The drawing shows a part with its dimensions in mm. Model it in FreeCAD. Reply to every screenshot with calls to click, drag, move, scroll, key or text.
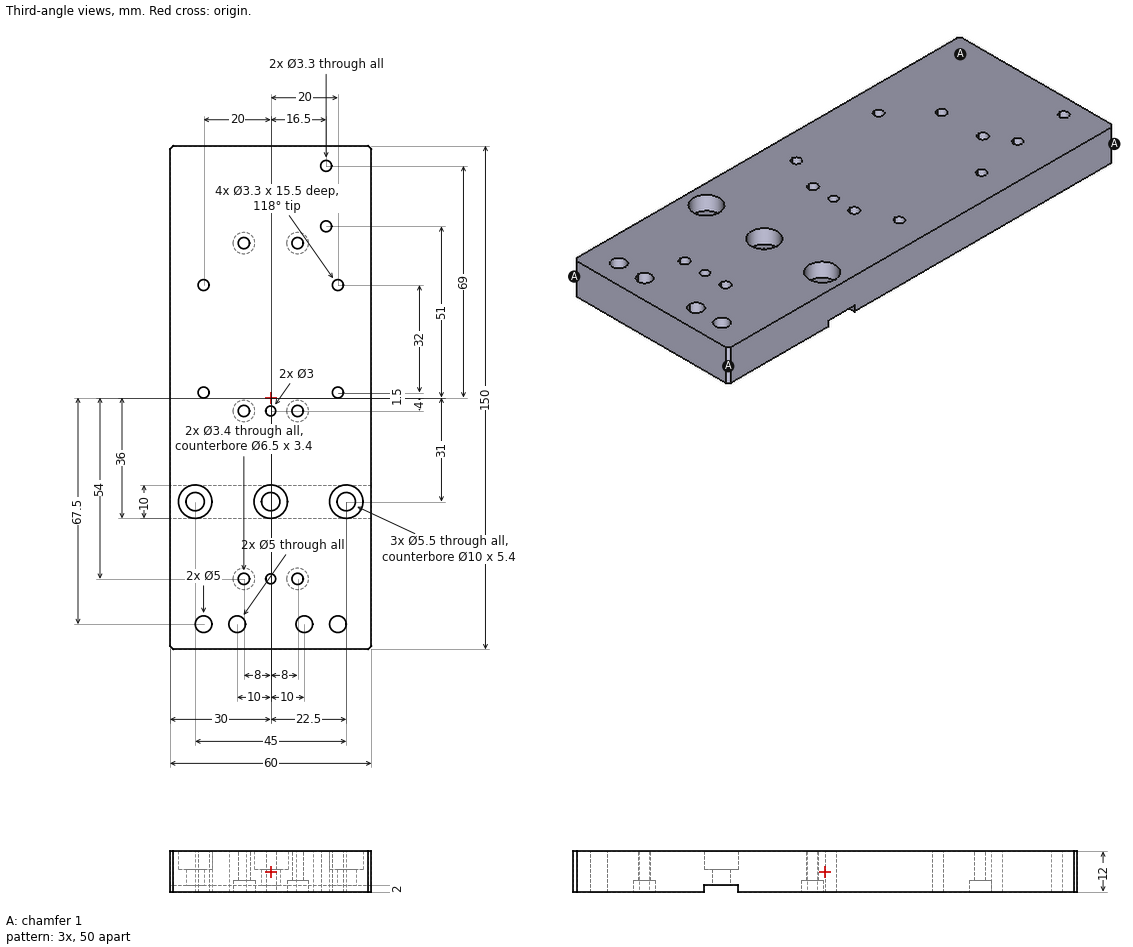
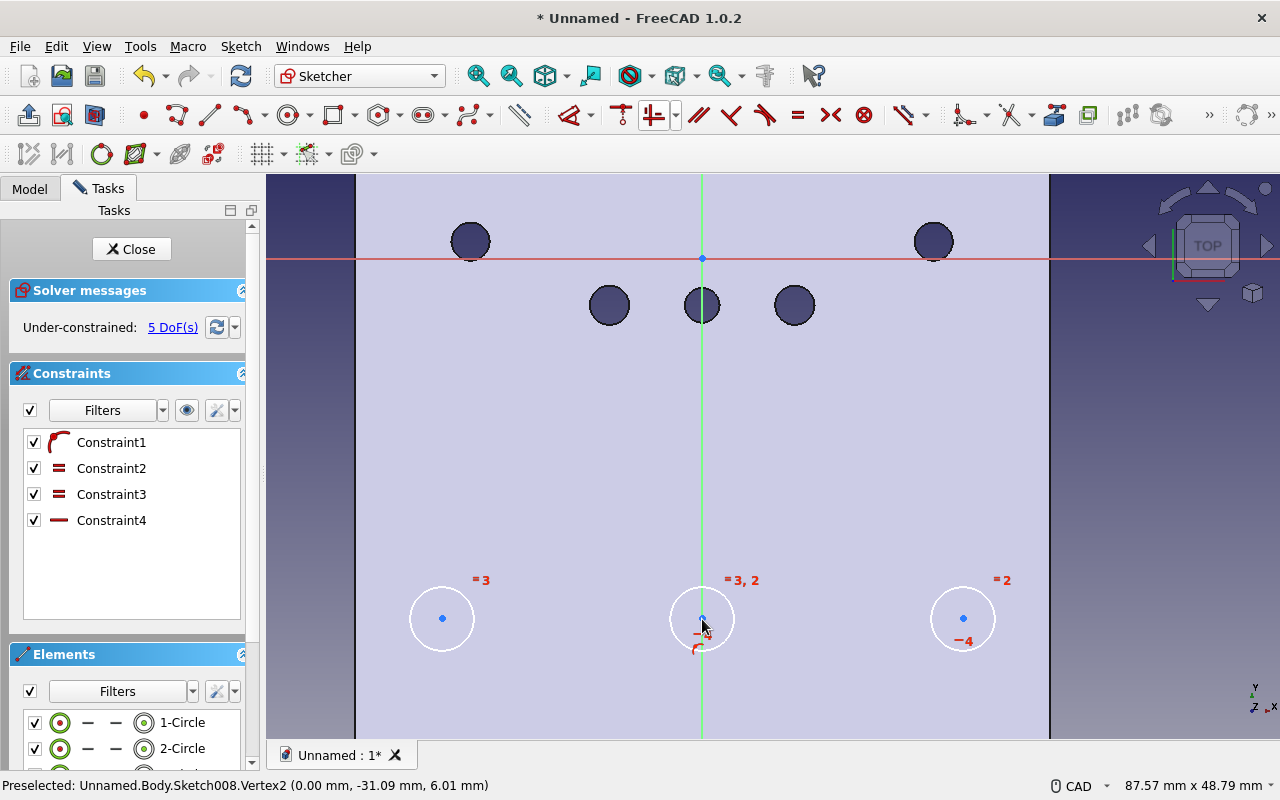
click(702, 619)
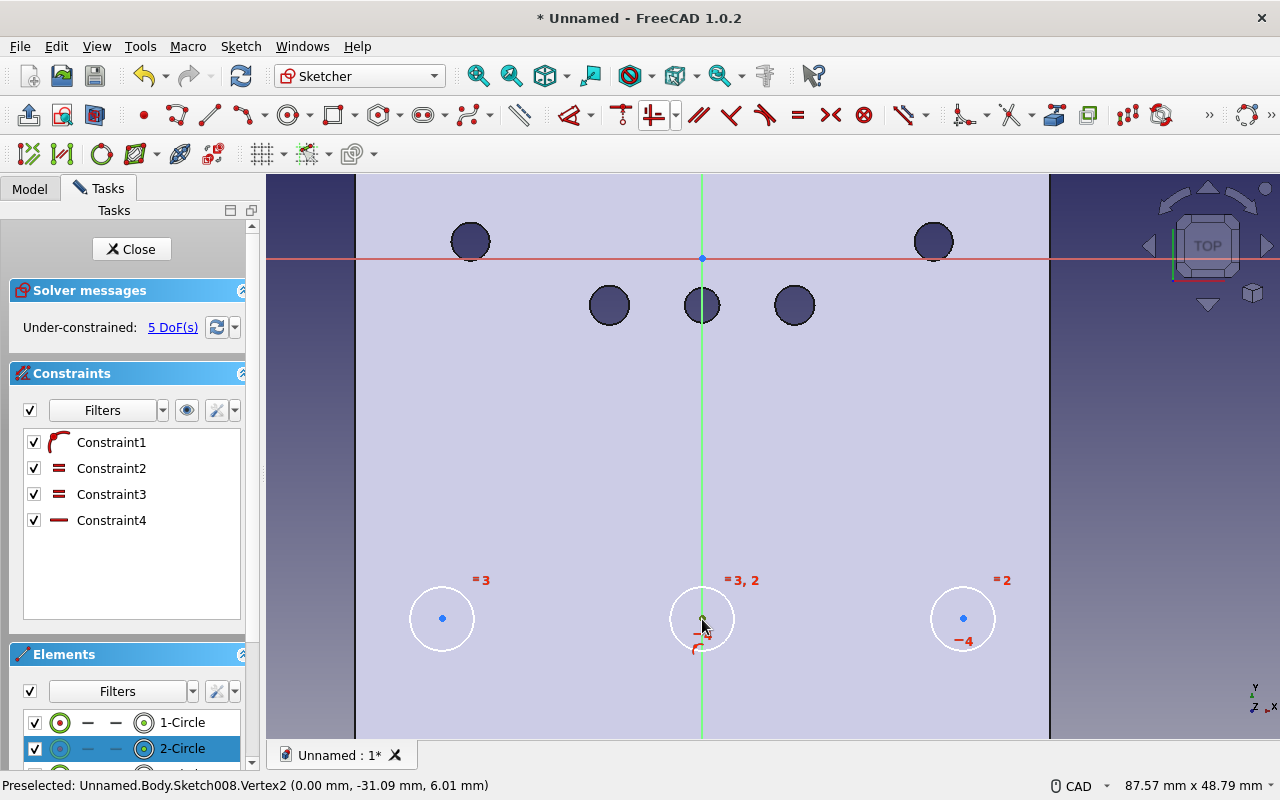
click(442, 619)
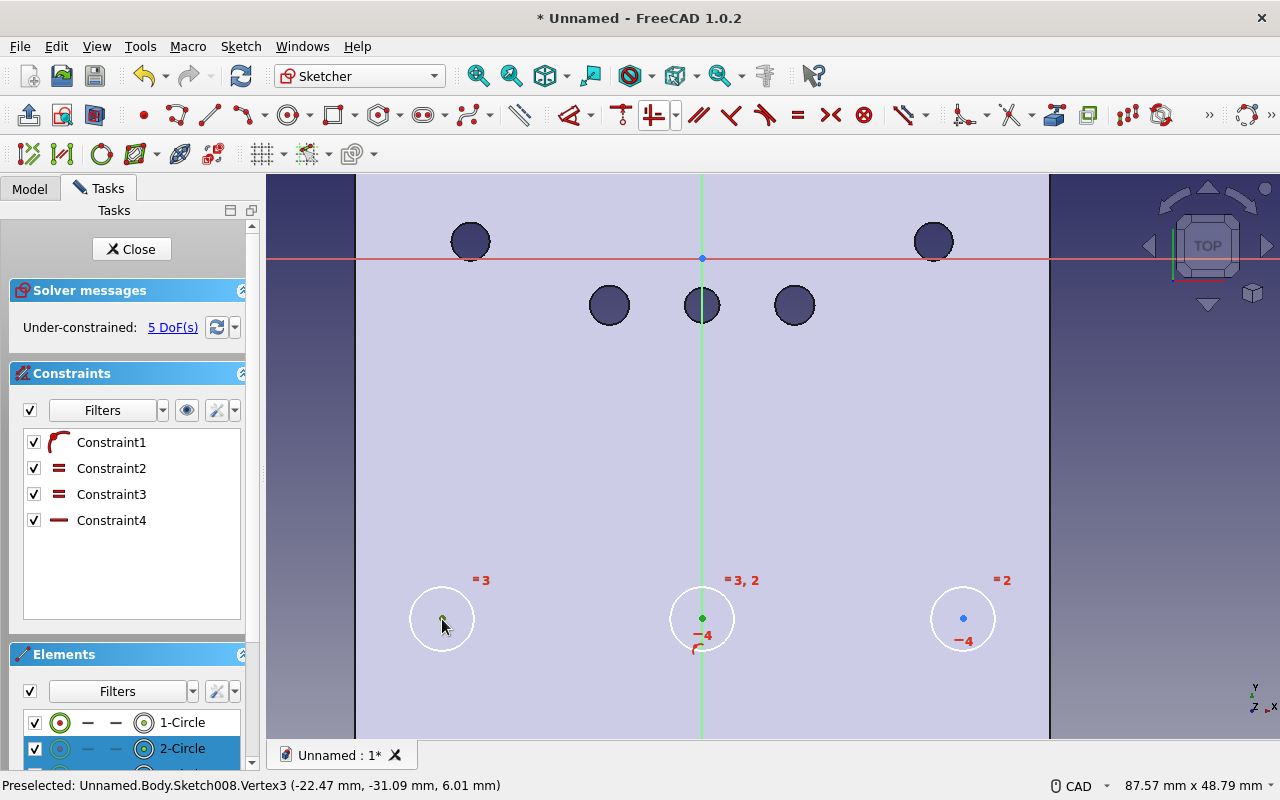
click(676, 116)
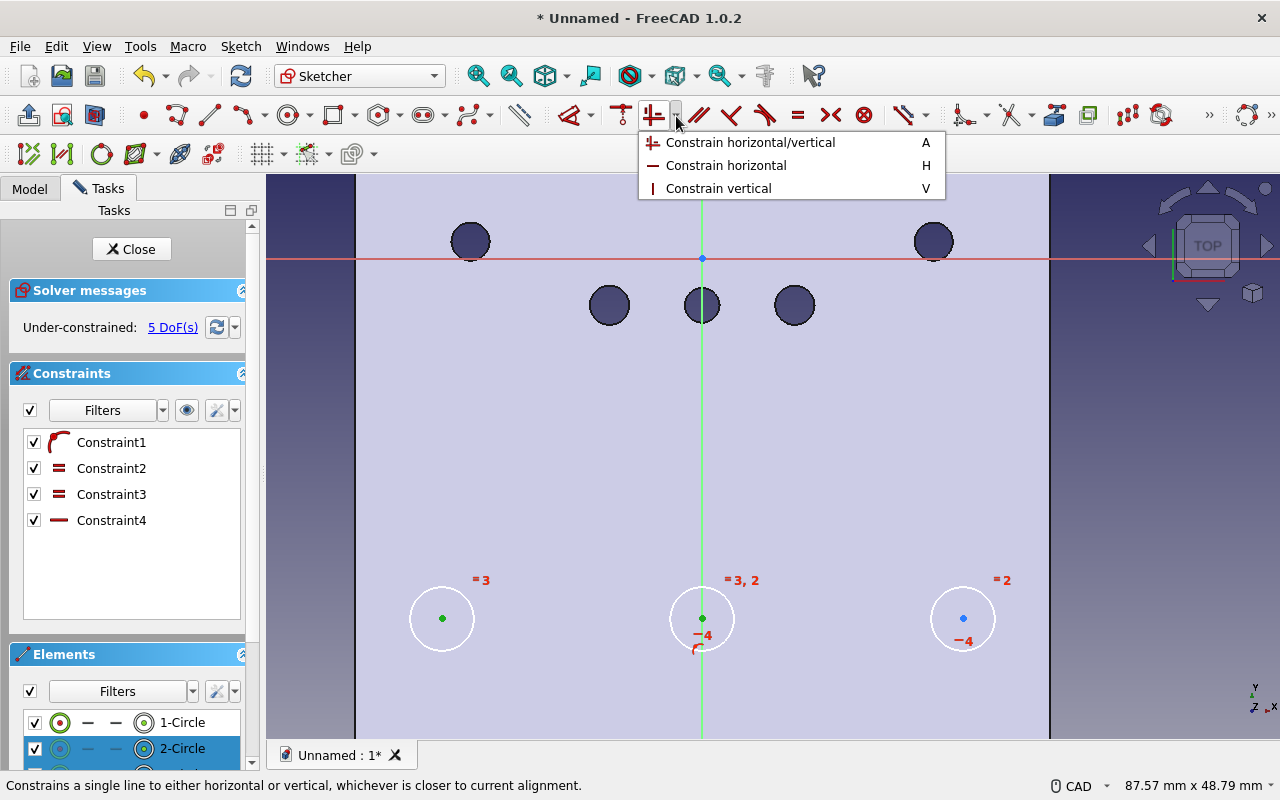
click(792, 166)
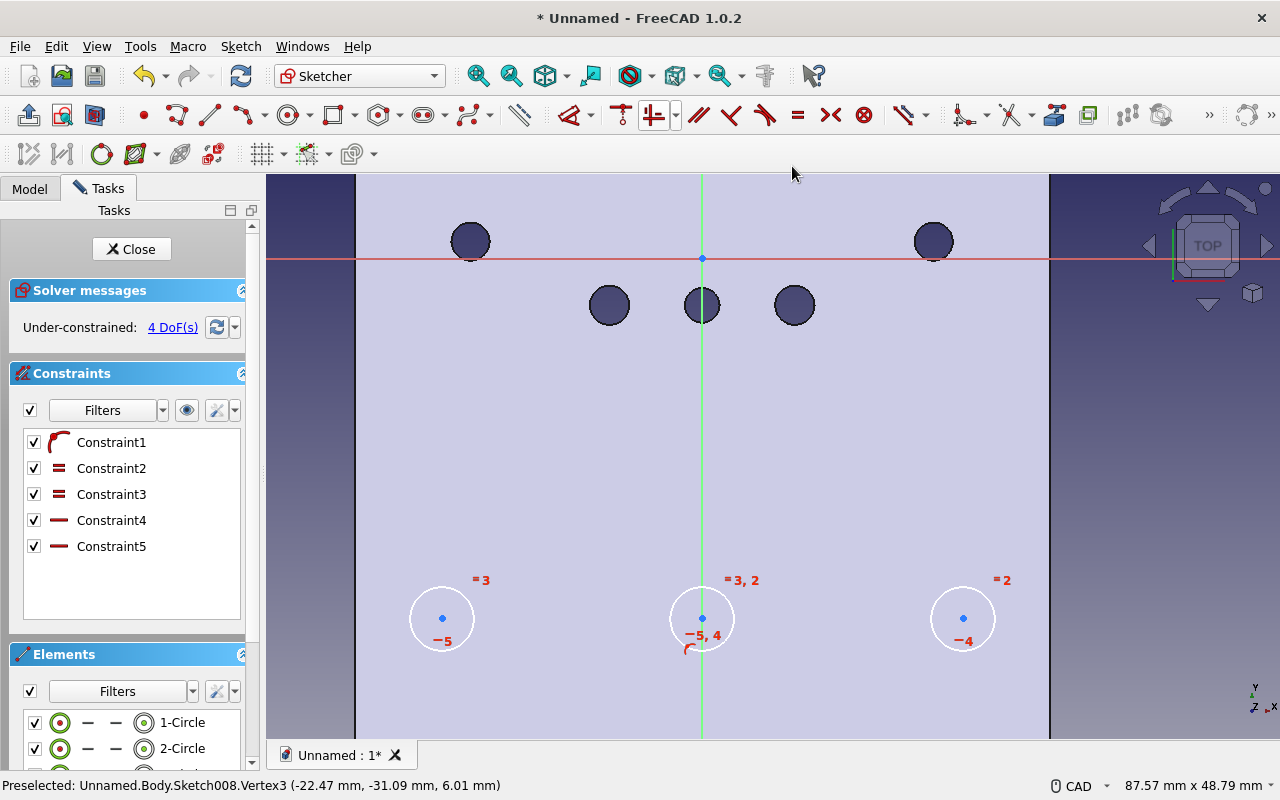
click(568, 116)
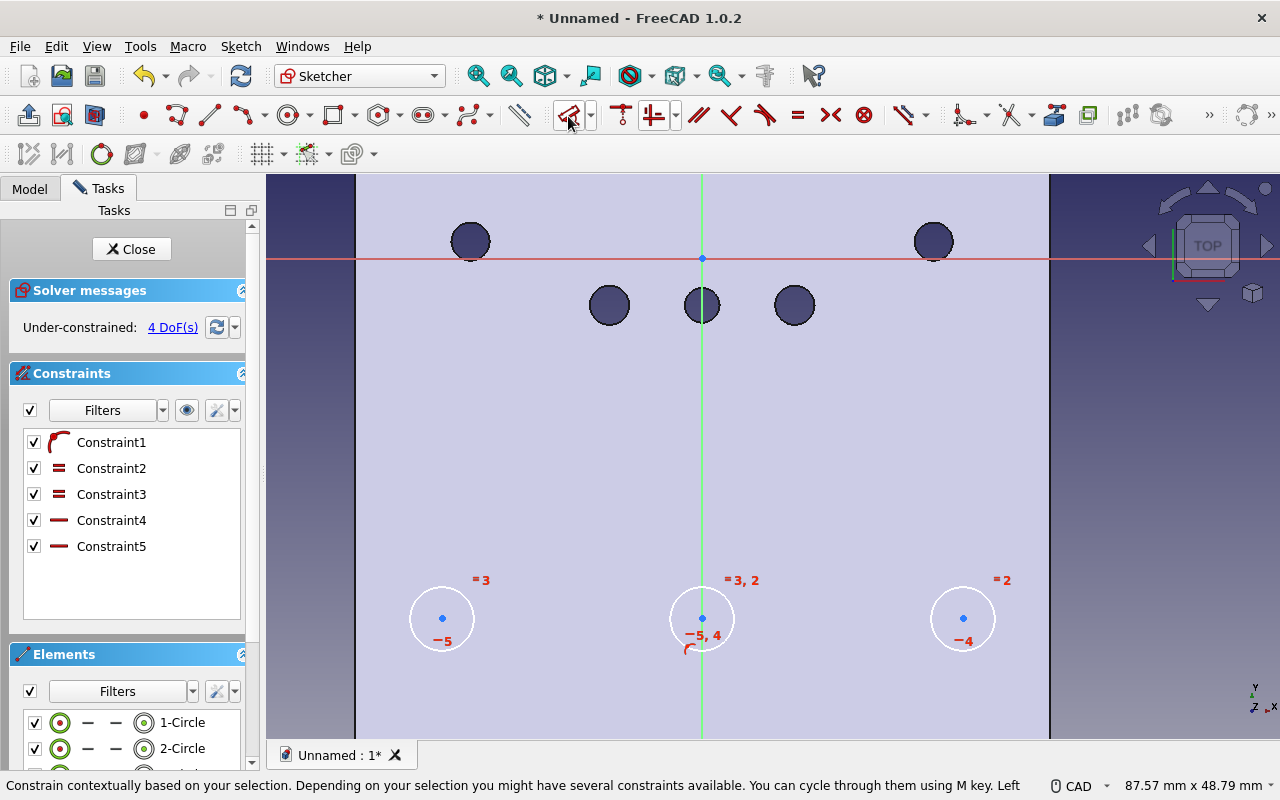
click(985, 596)
click(1007, 573)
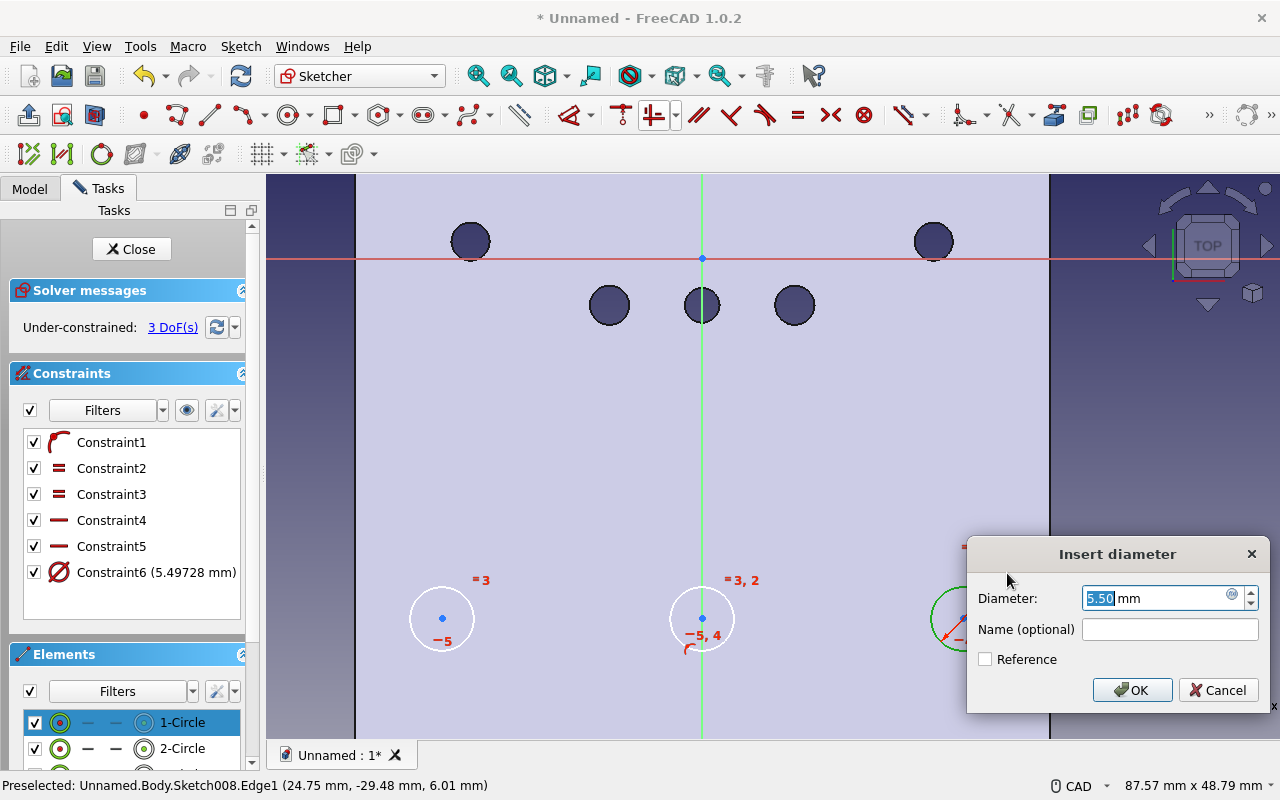
text(5.5)
key(Return)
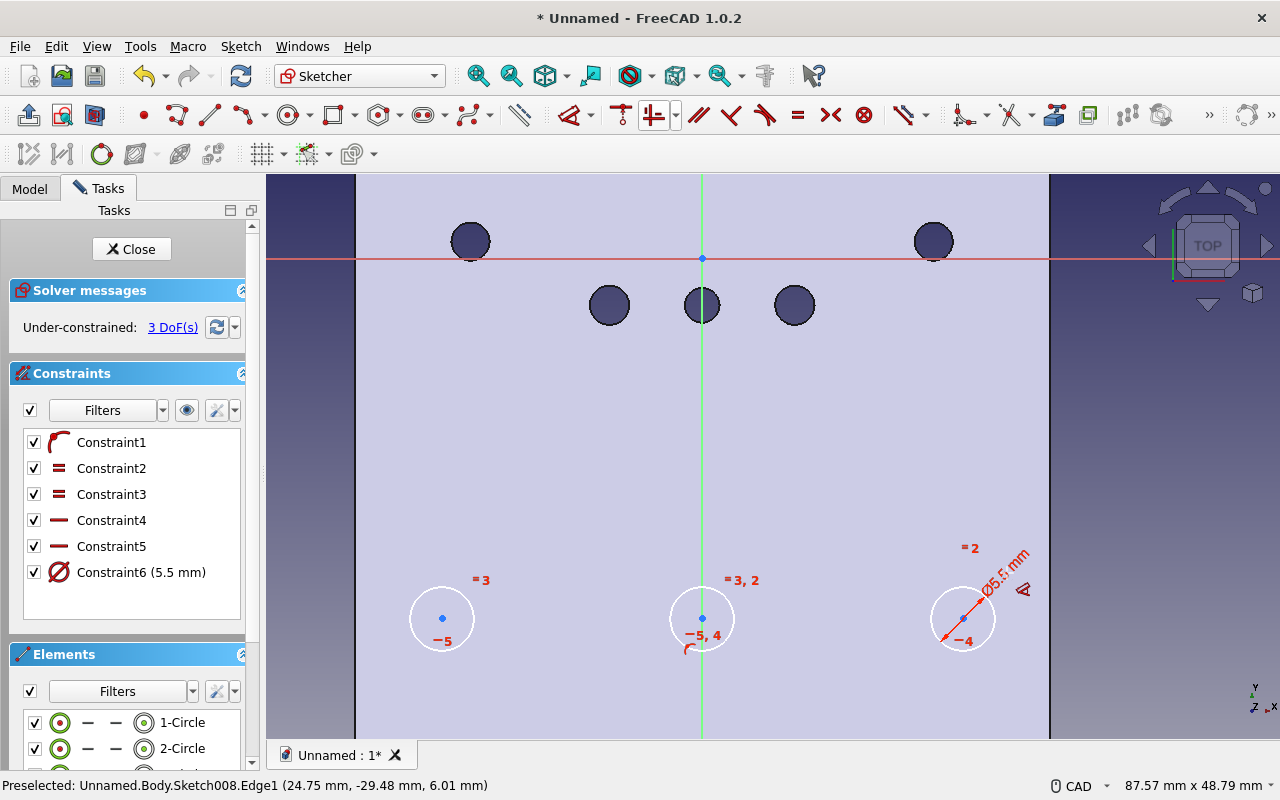
click(963, 619)
click(997, 439)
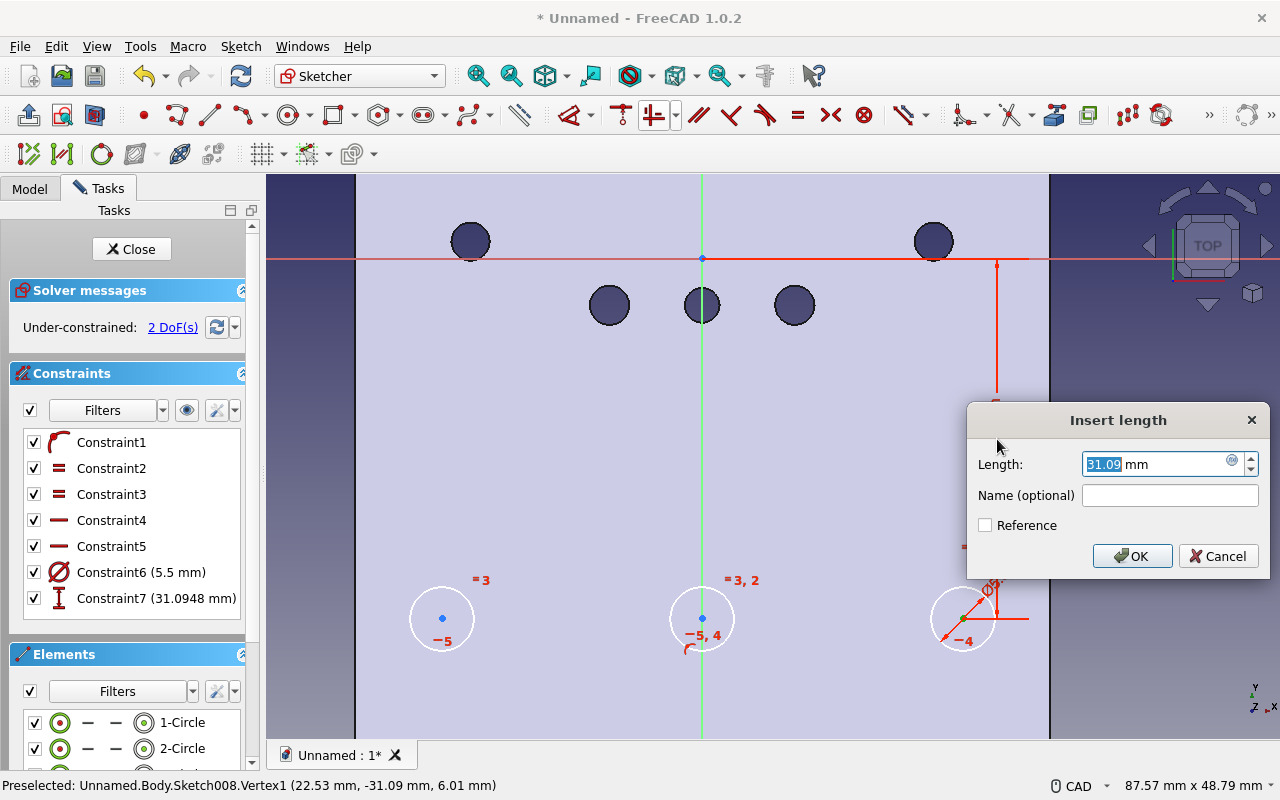
text(31)
key(Return)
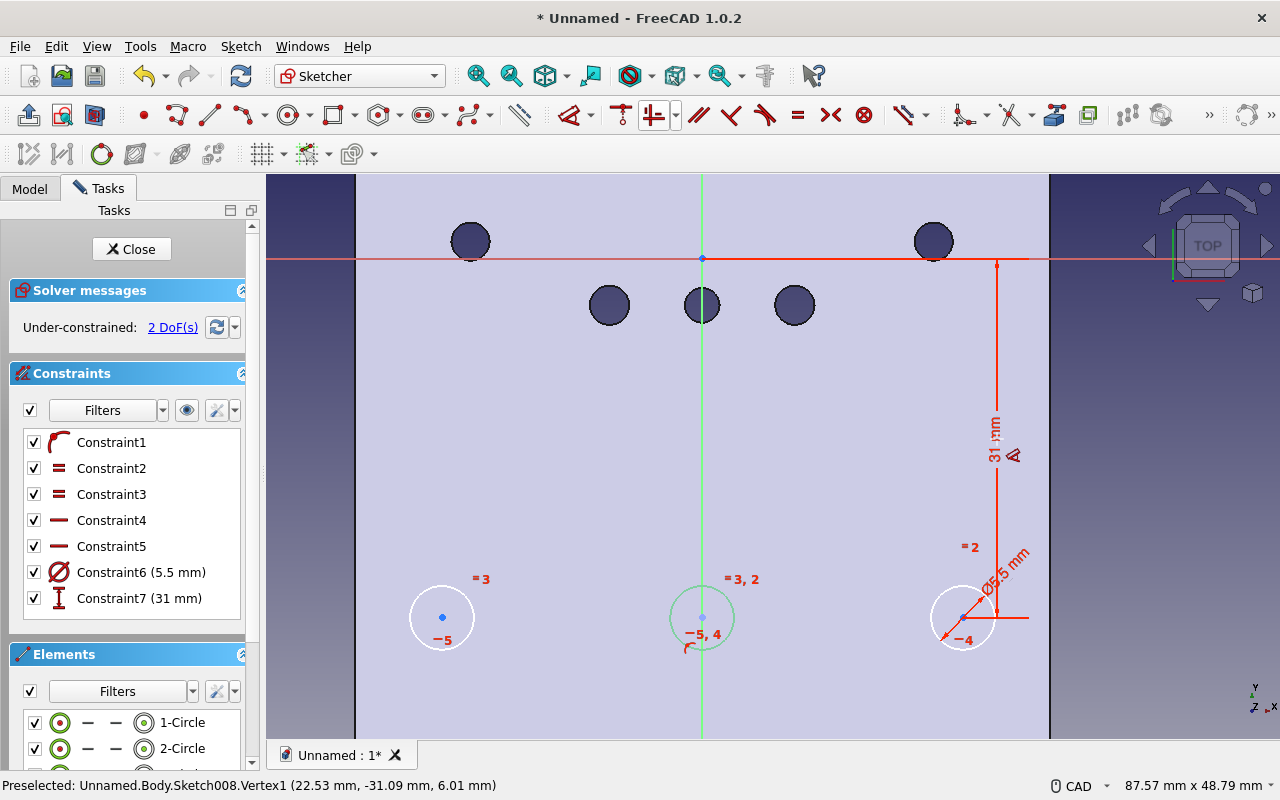
click(963, 618)